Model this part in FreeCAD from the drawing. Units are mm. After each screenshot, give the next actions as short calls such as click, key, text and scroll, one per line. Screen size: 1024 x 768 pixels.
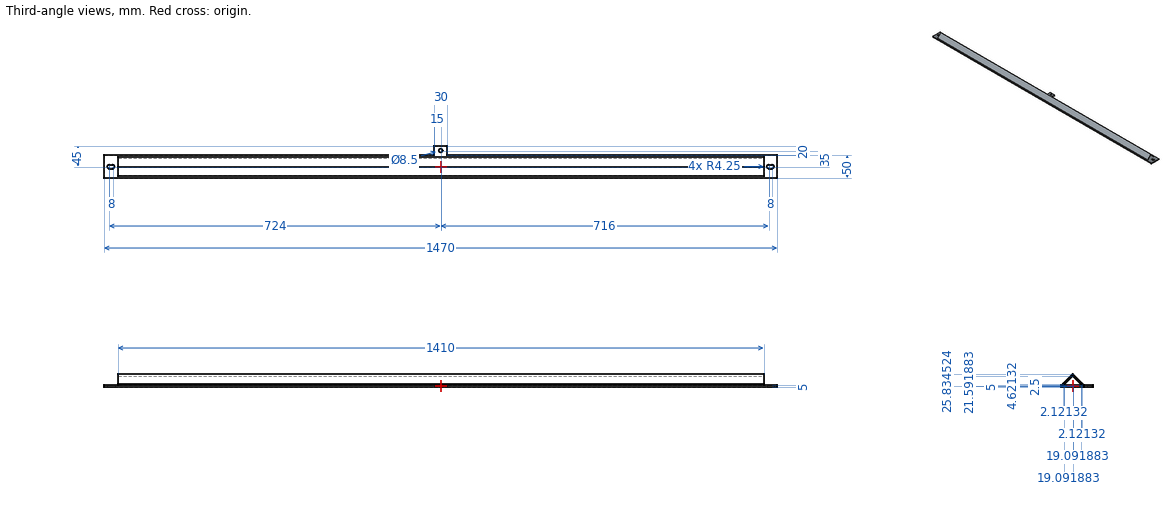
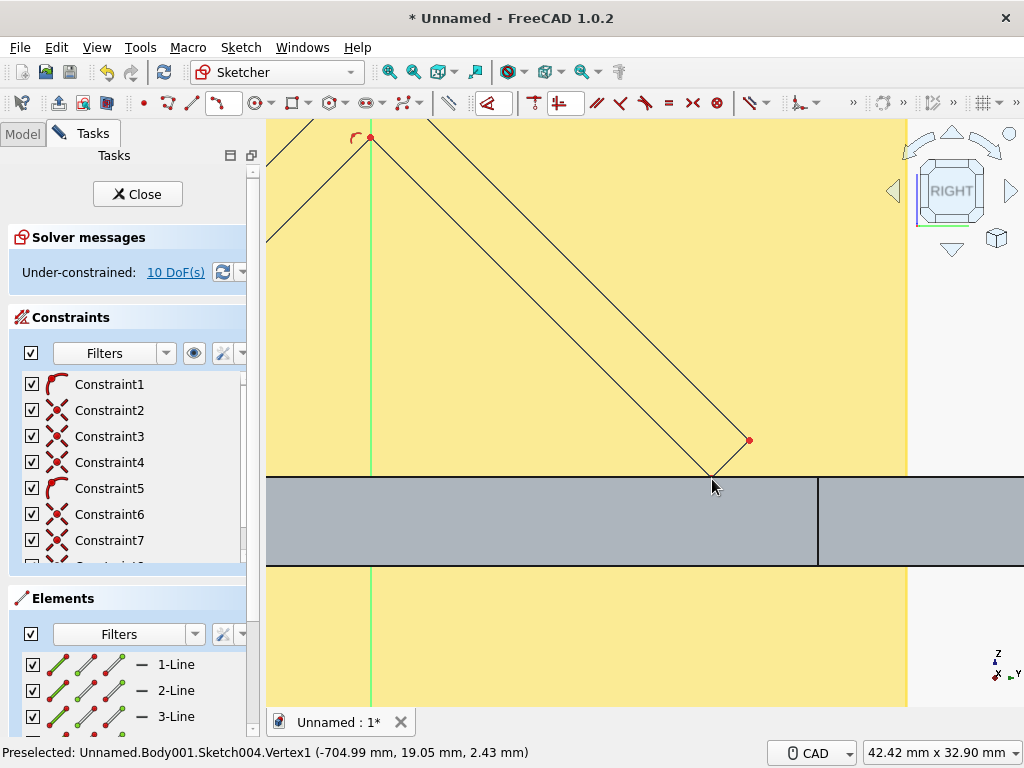
click(711, 478)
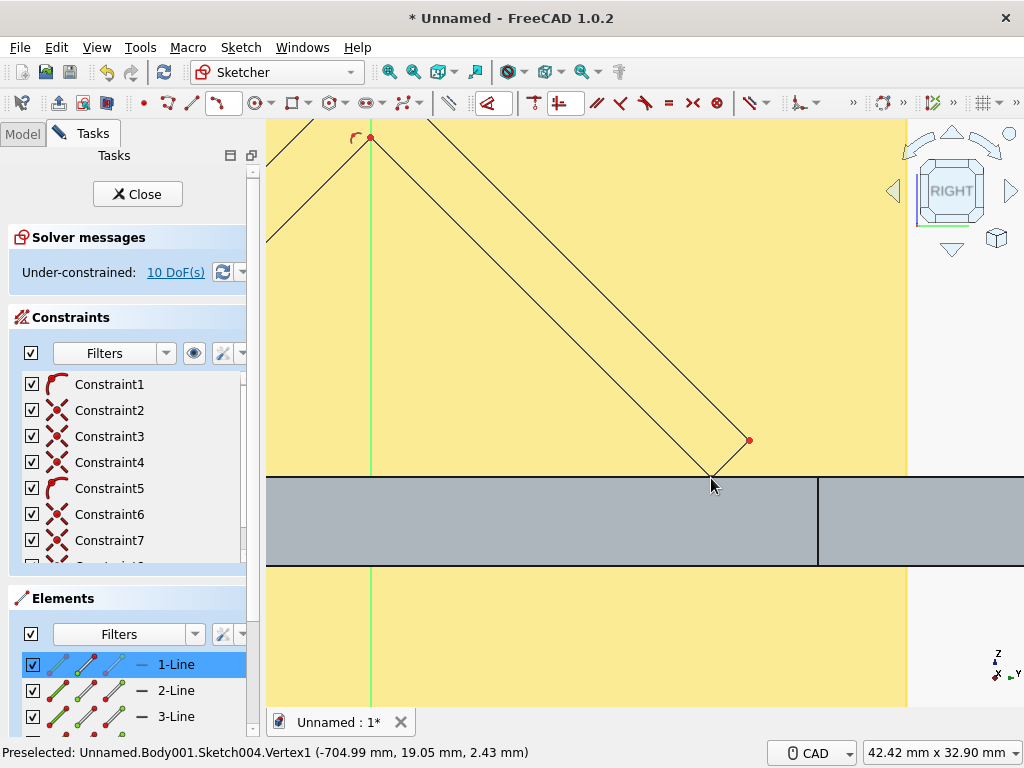
key(i)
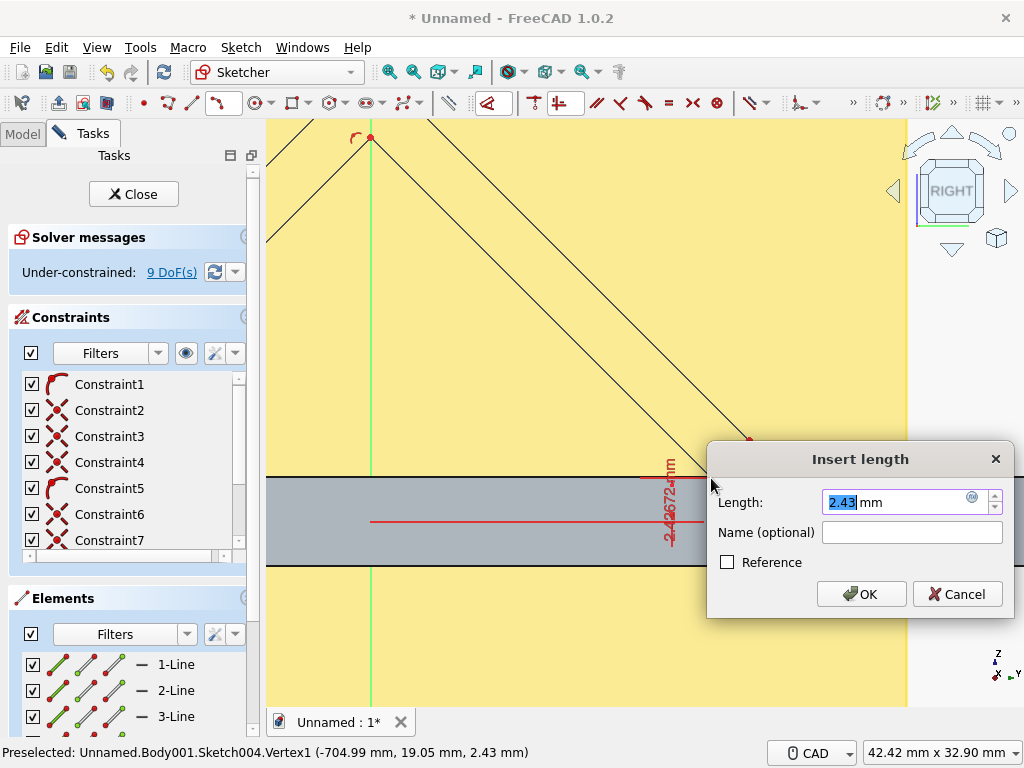
text(2.5)
key(Return)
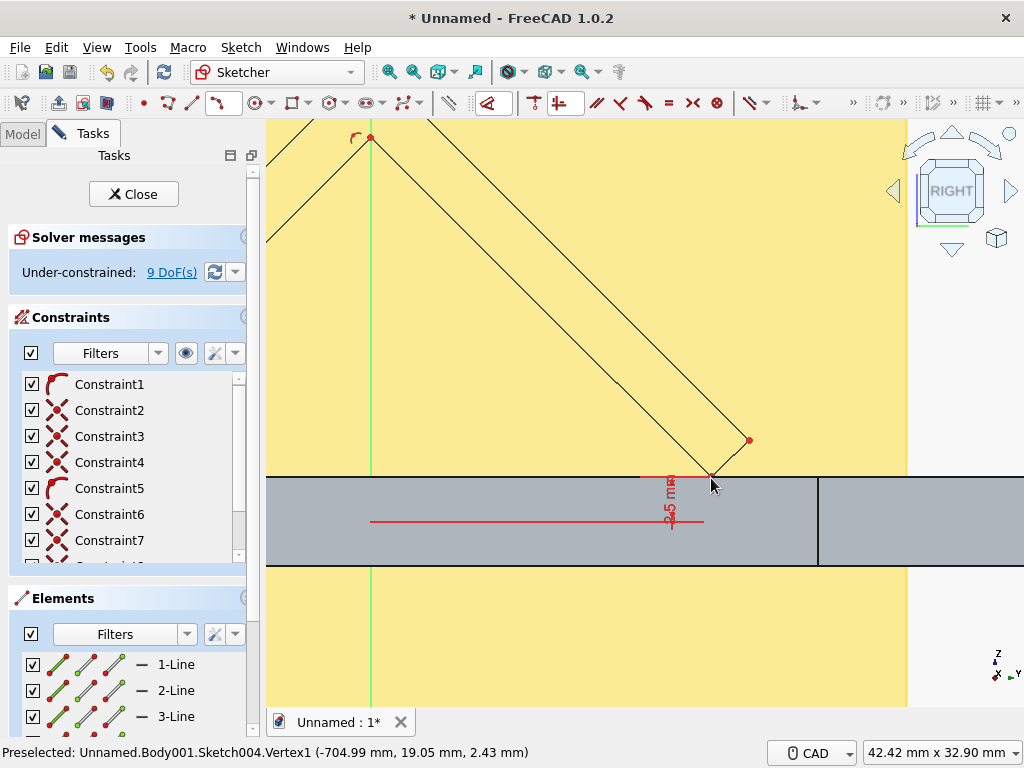
scroll(827, 562, down, 3)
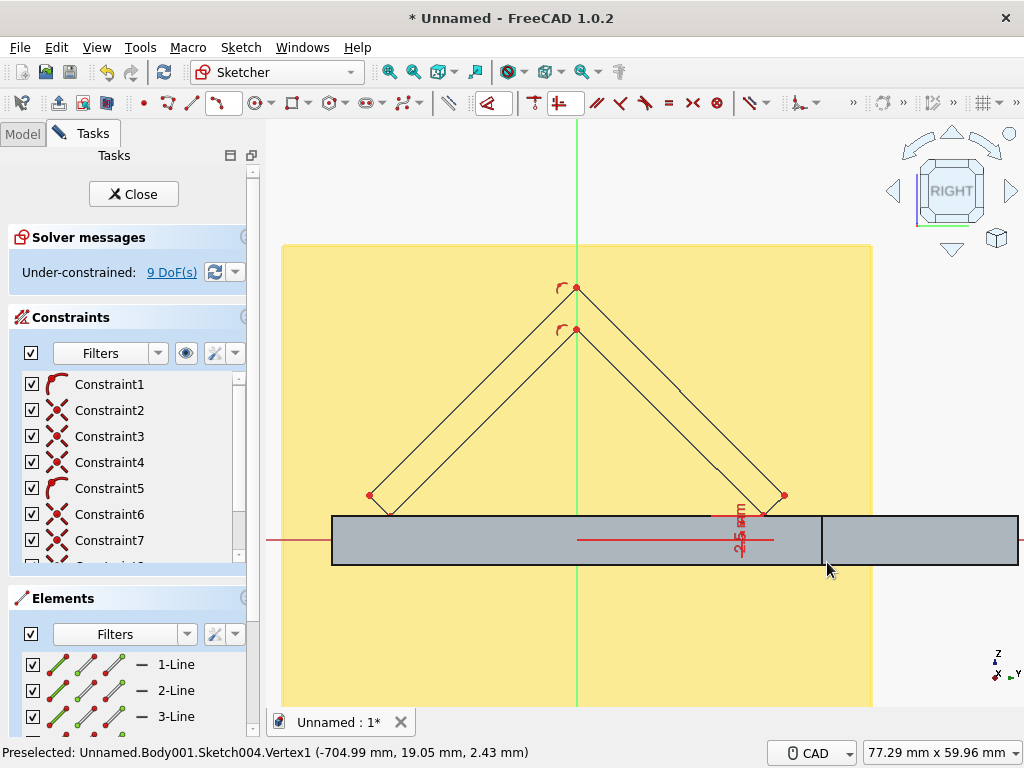
scroll(390, 516, up, 3)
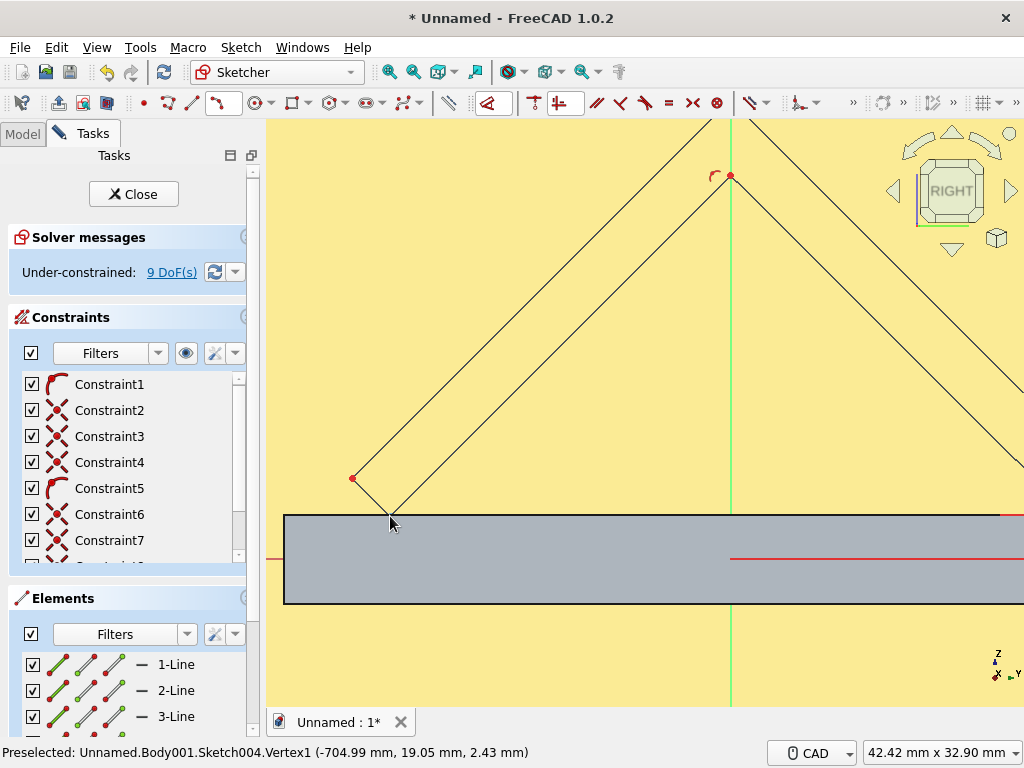
click(390, 516)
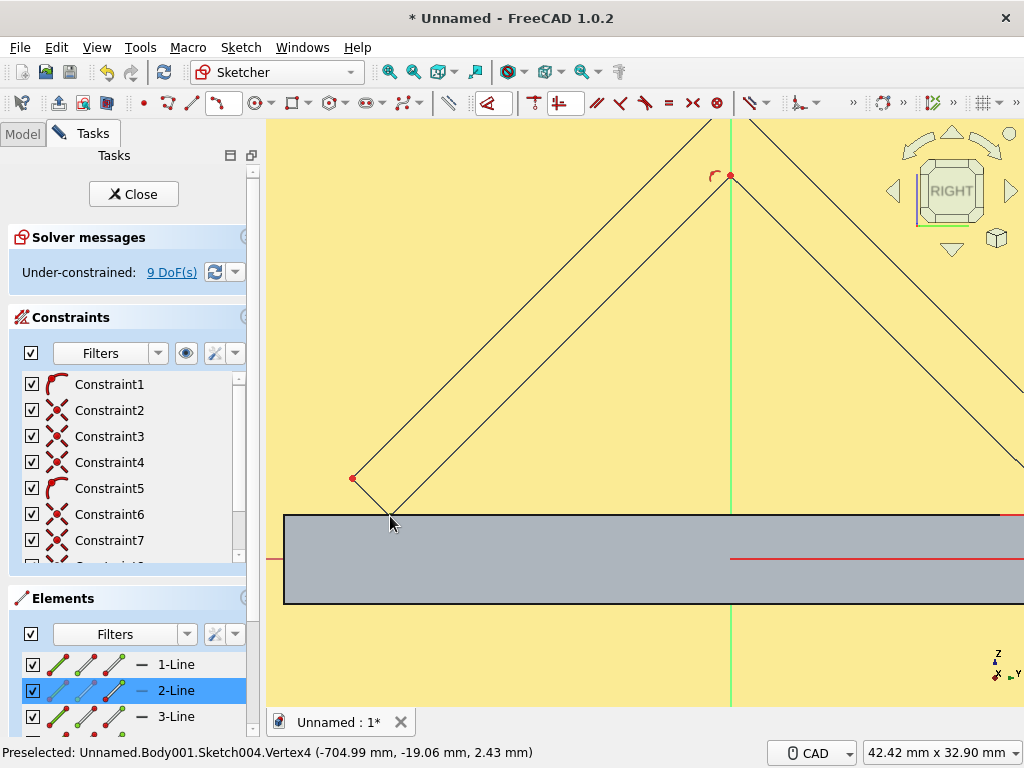
click(506, 104)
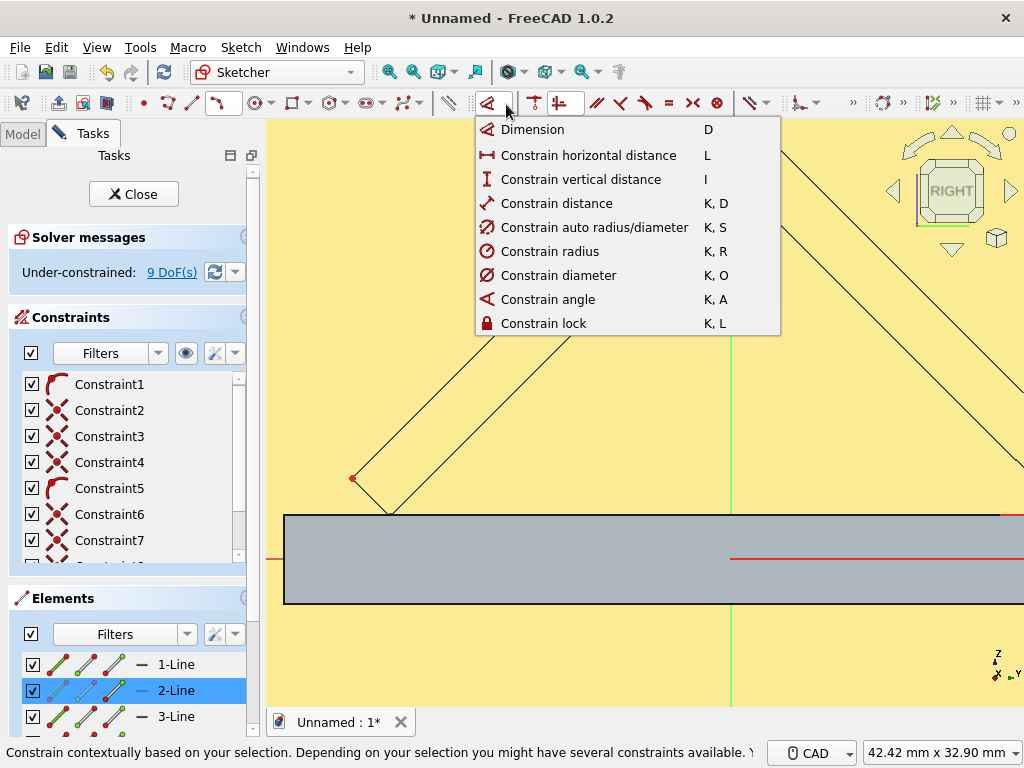
click(628, 179)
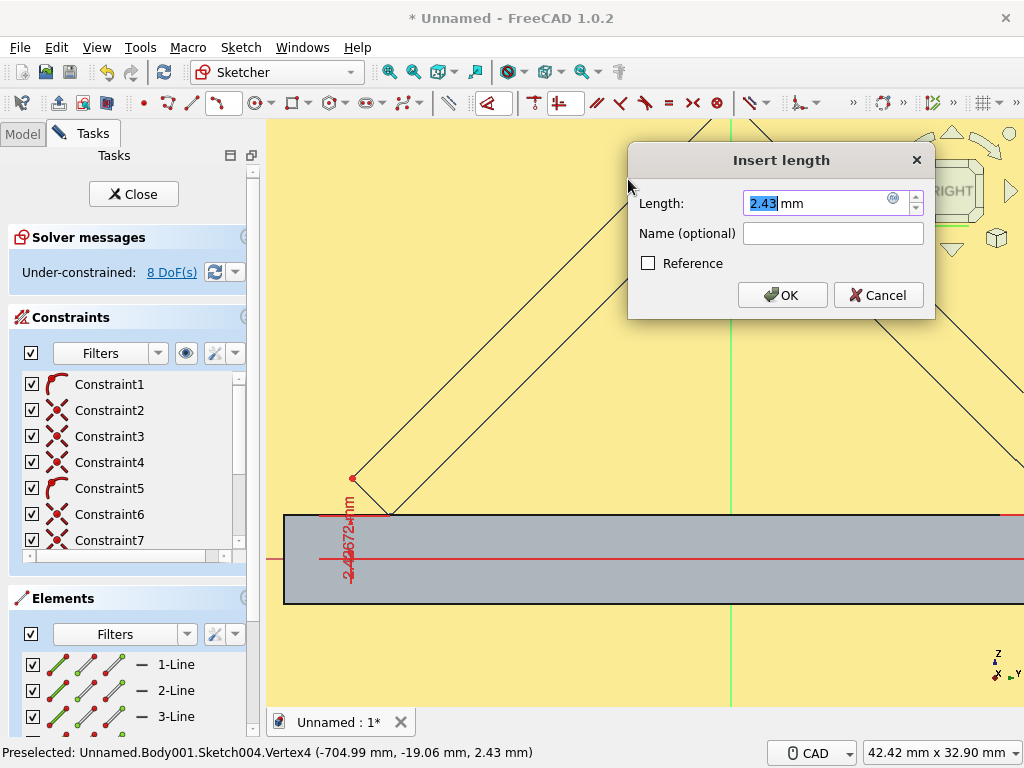
text(2.5)
key(Return)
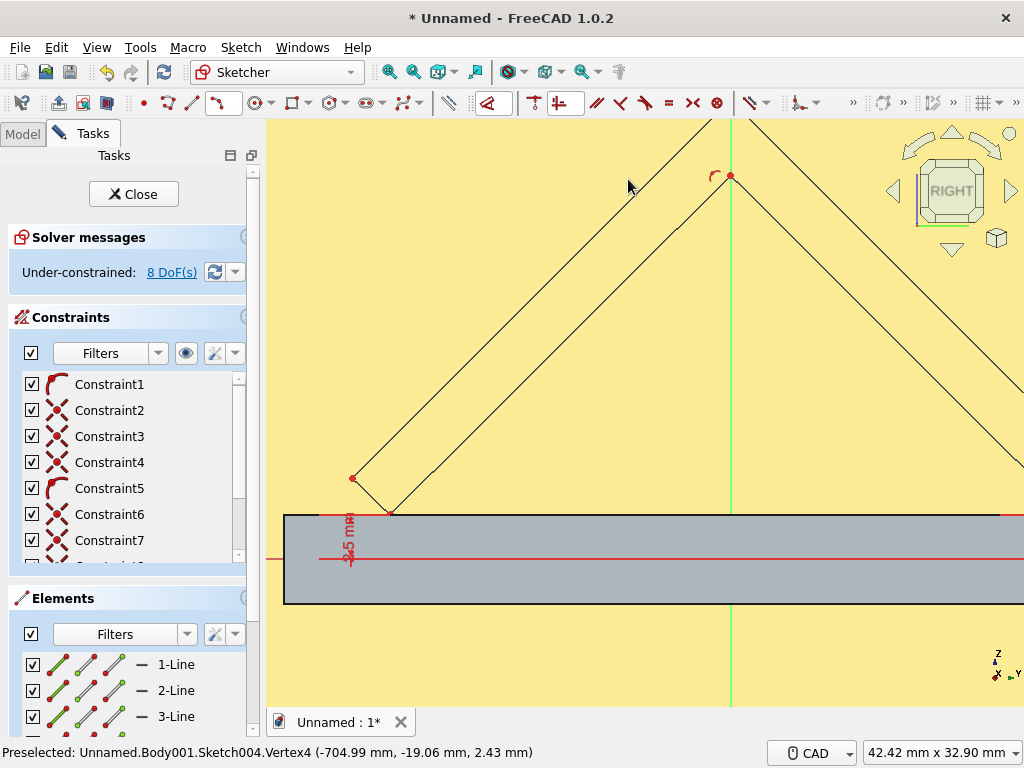
click(352, 478)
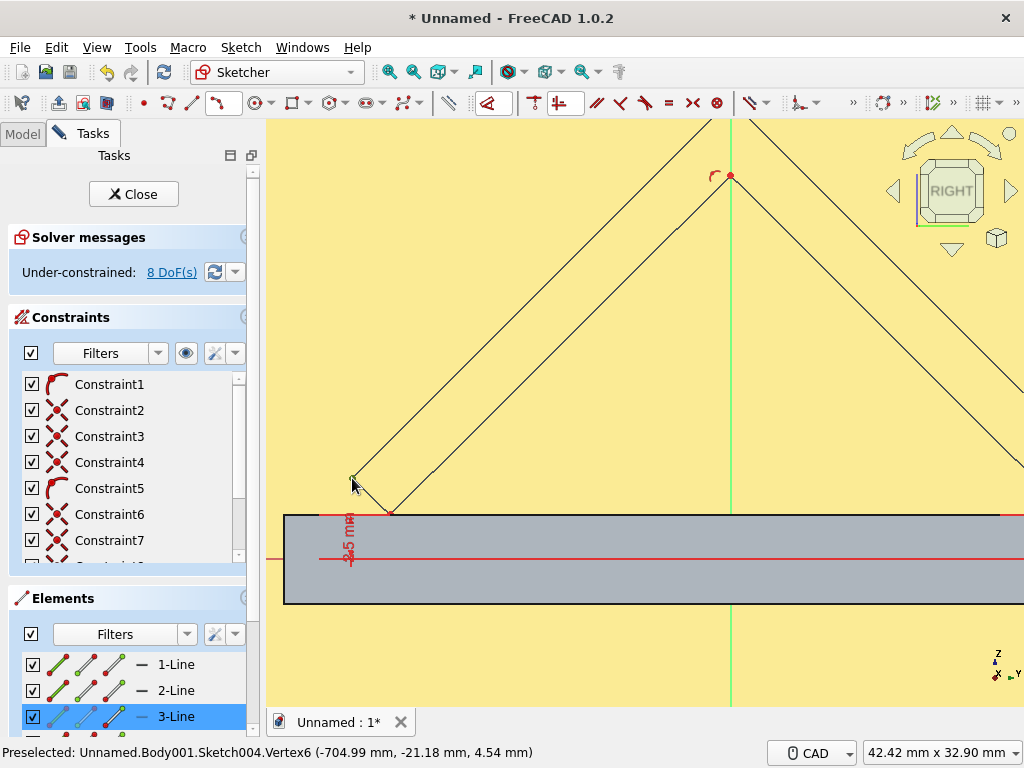
click(506, 104)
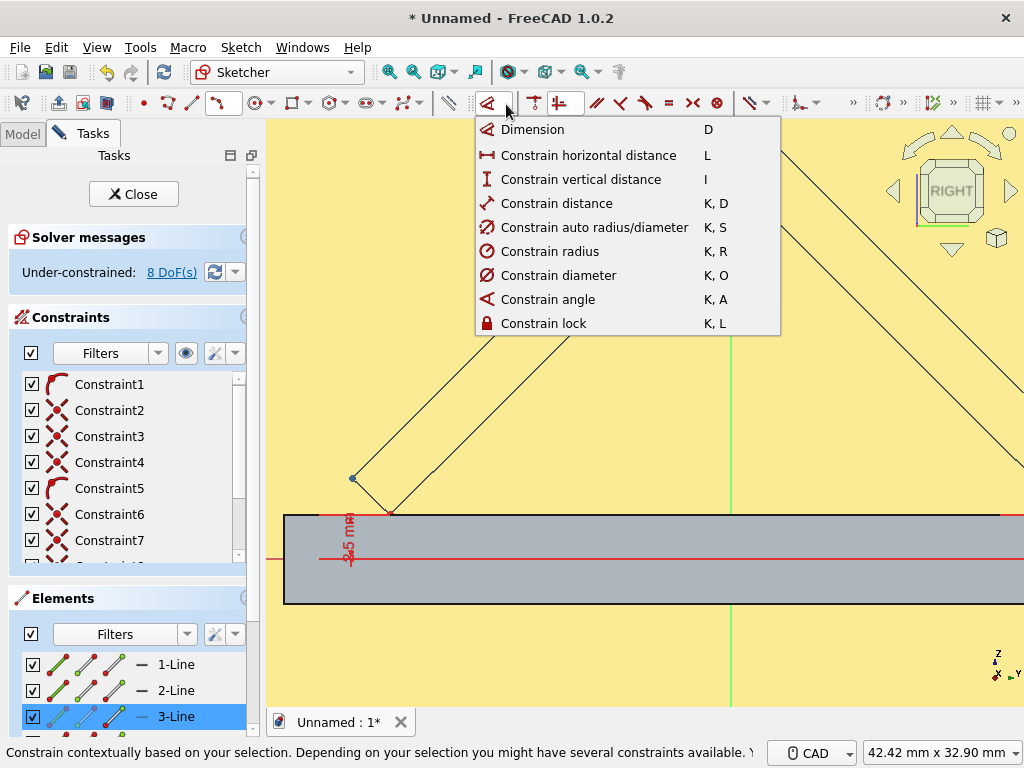
click(628, 179)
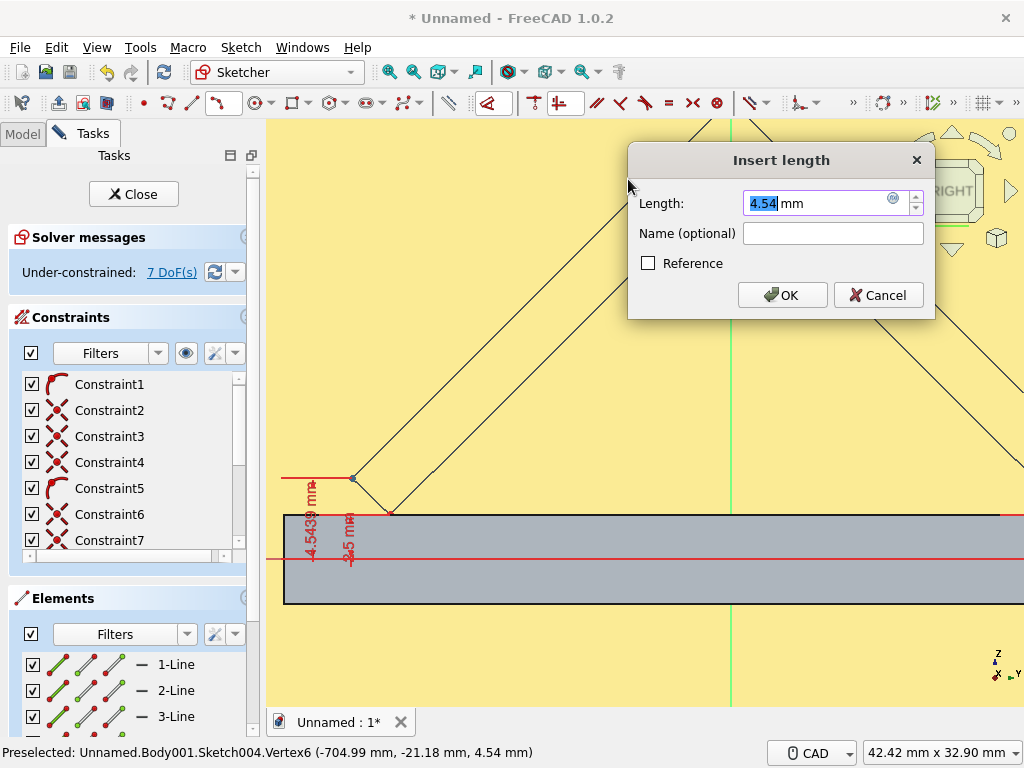
text(4.62132)
key(Return)